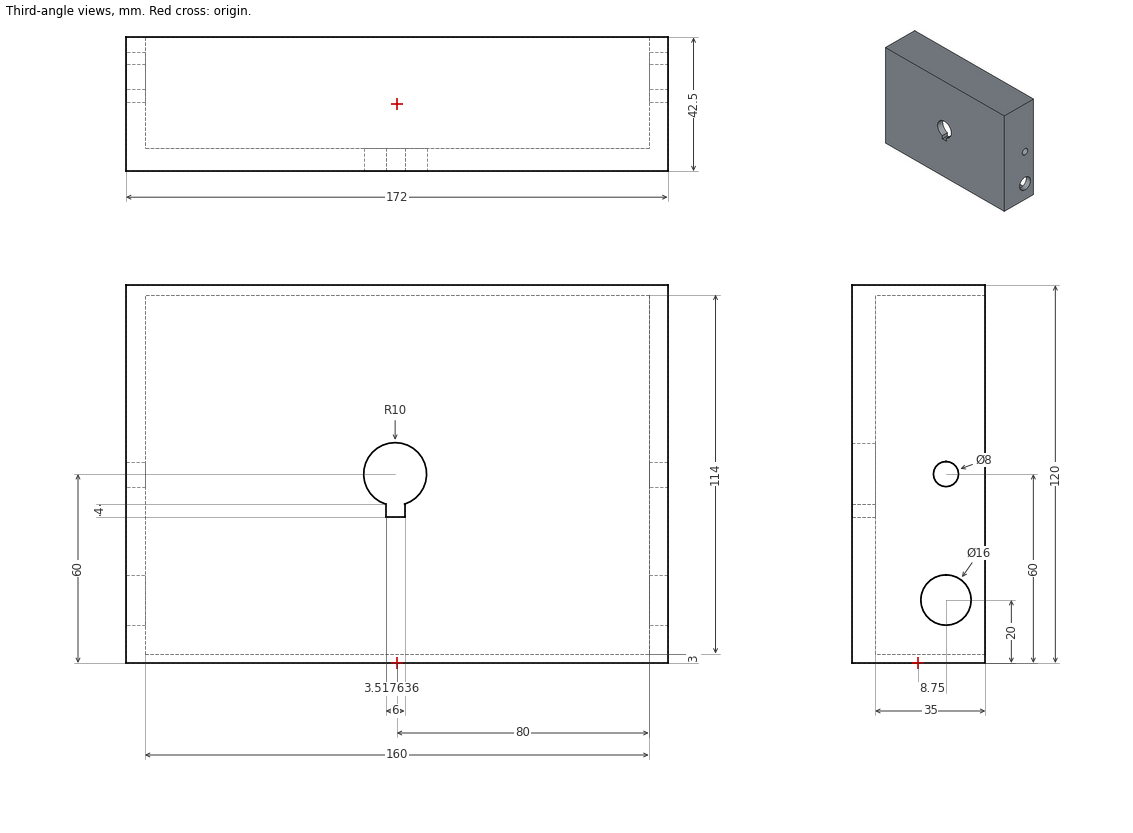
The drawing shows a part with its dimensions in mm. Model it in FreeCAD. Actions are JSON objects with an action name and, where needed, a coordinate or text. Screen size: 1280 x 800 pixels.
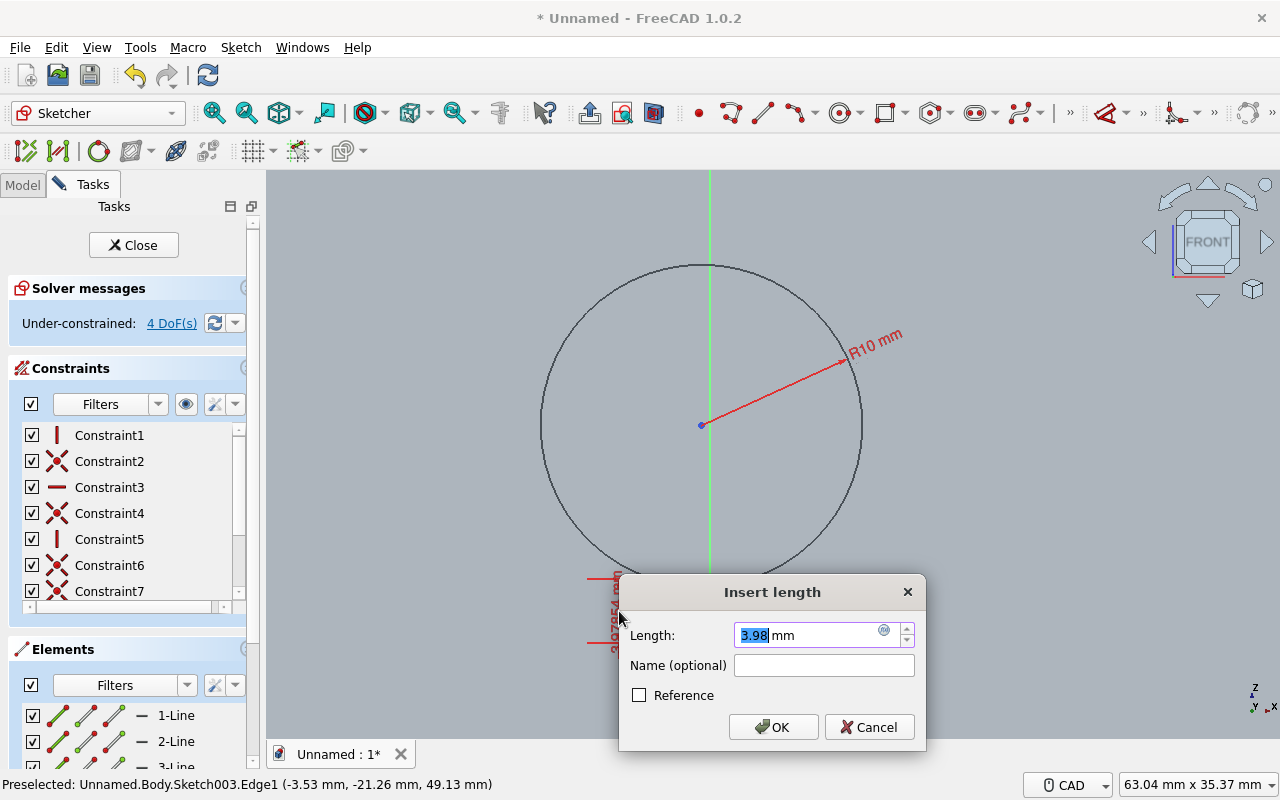
{"action": "type", "text": "4"}
{"action": "key", "text": "Return"}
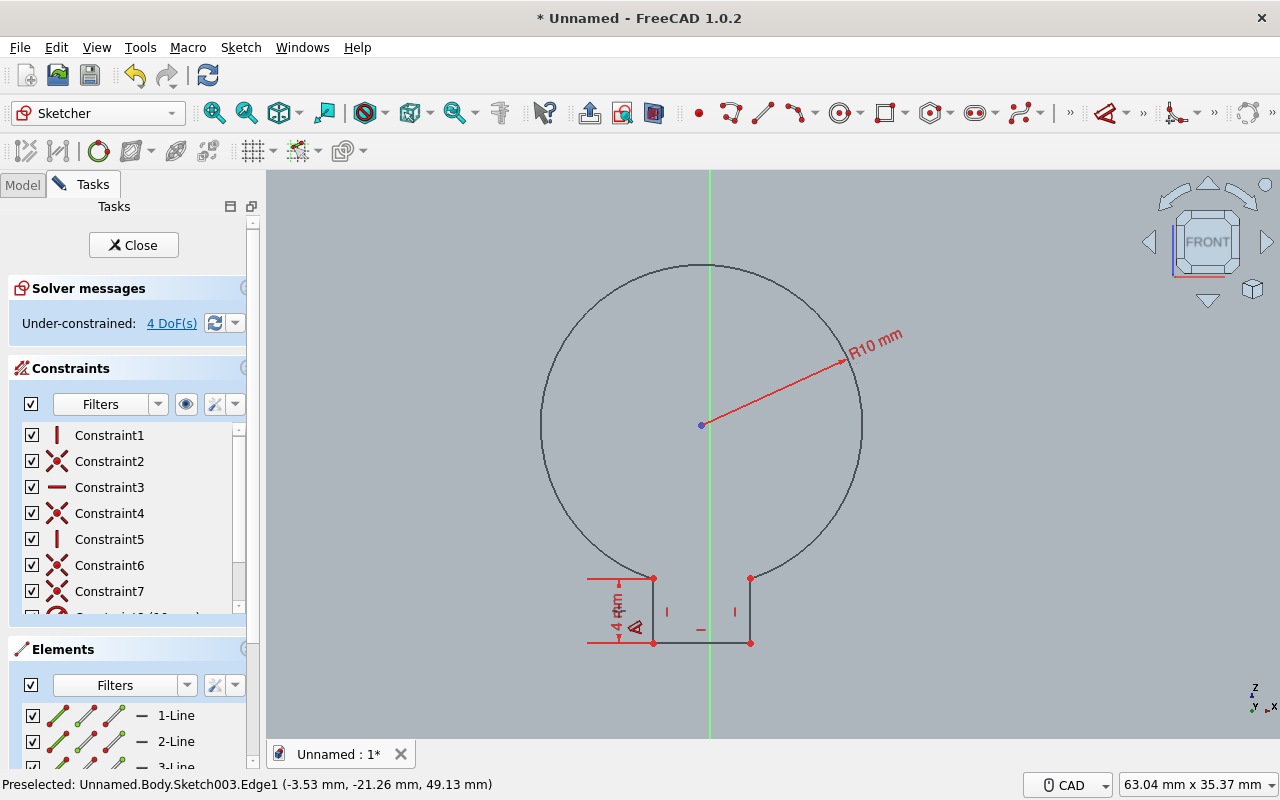
{"action": "left_click", "coordinate": [682, 643]}
{"action": "left_click", "coordinate": [679, 677]}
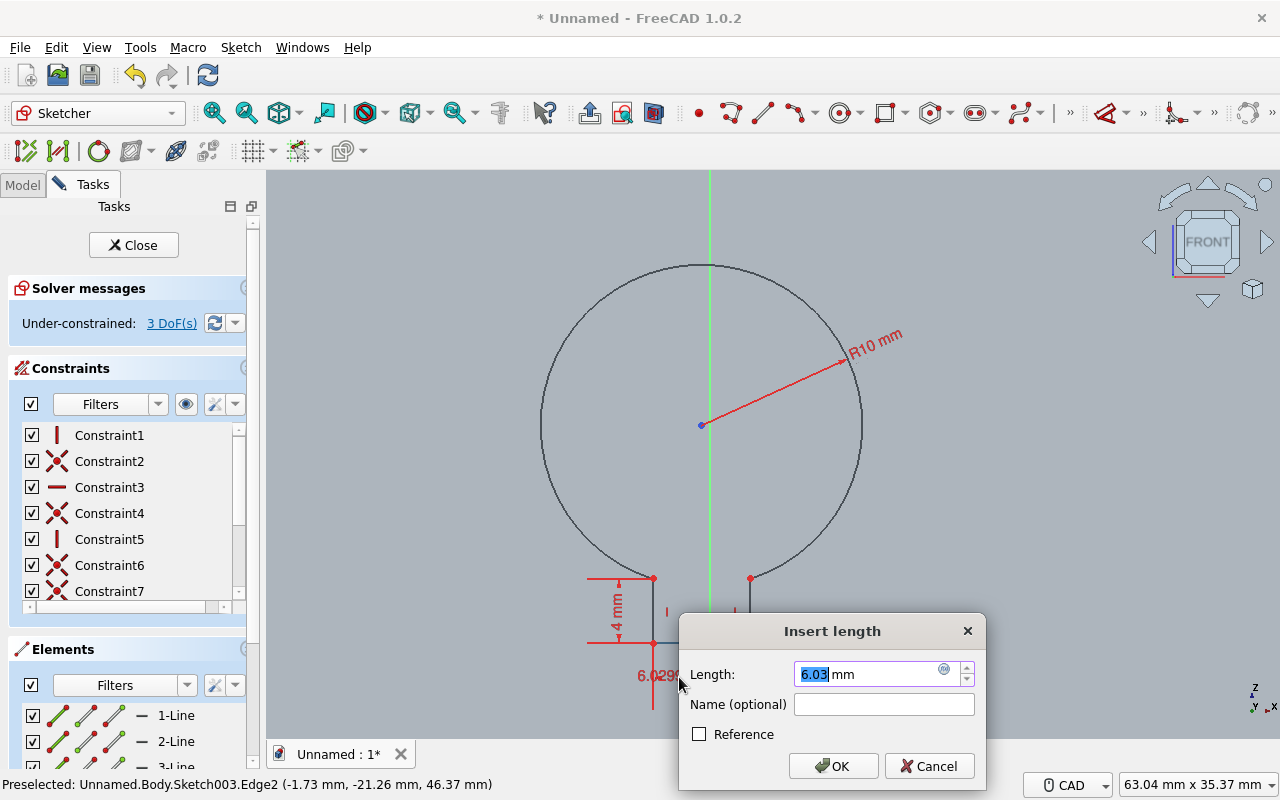
{"action": "type", "text": "6"}
{"action": "key", "text": "Return"}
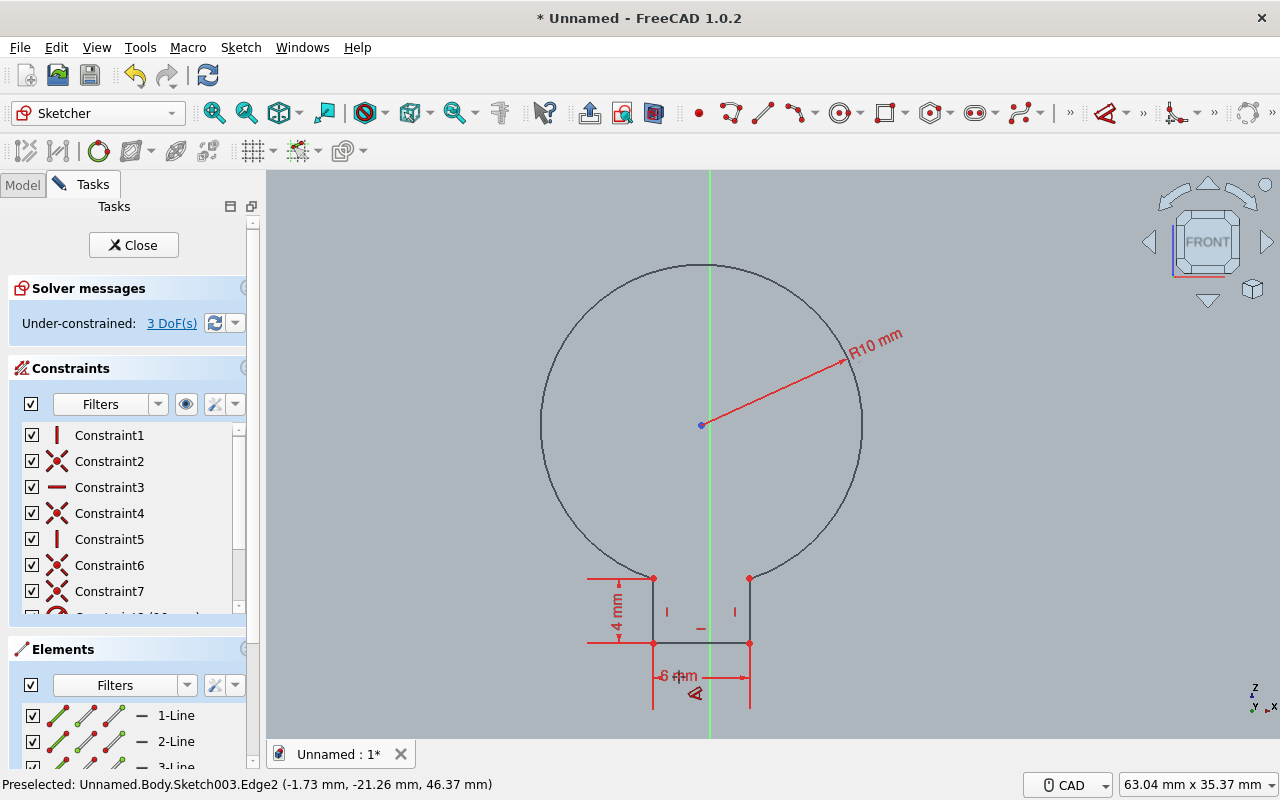
{"action": "left_click", "coordinate": [750, 624]}
{"action": "left_click", "coordinate": [784, 611]}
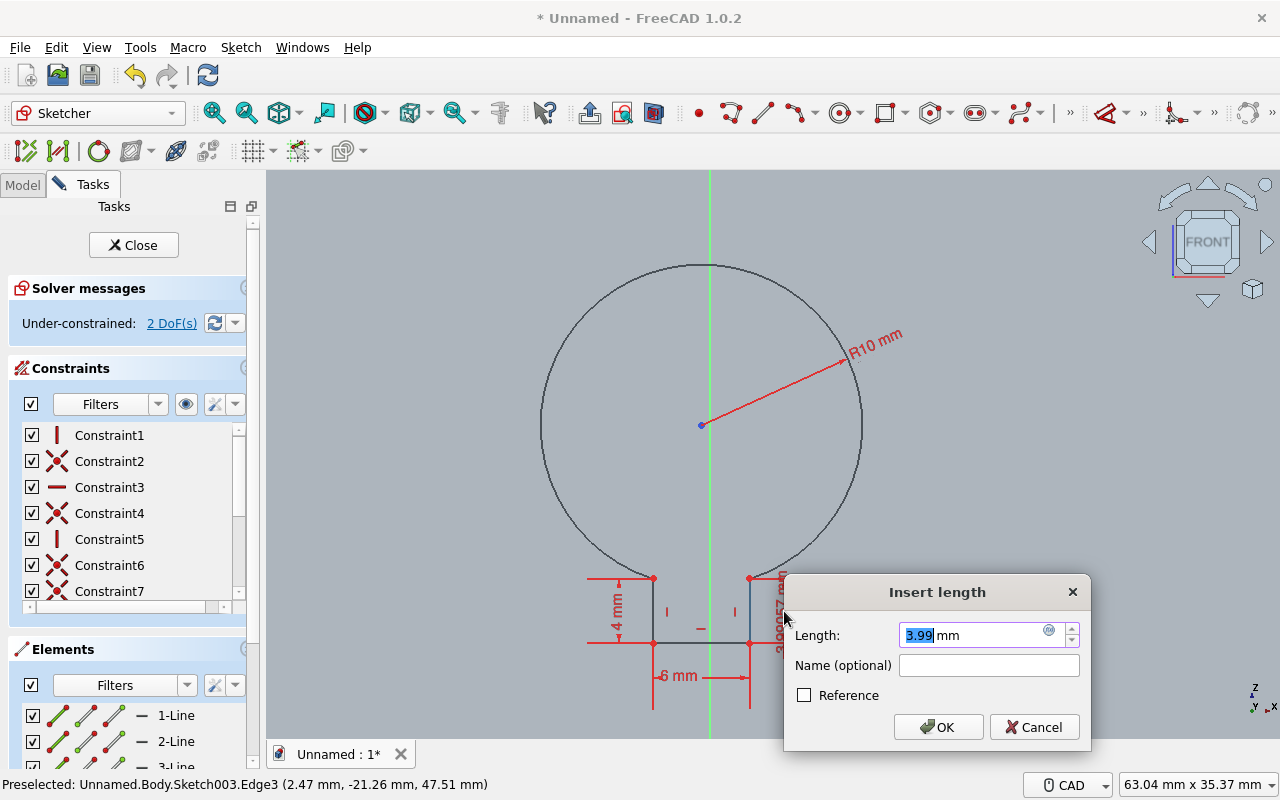
{"action": "type", "text": "4"}
{"action": "key", "text": "Return"}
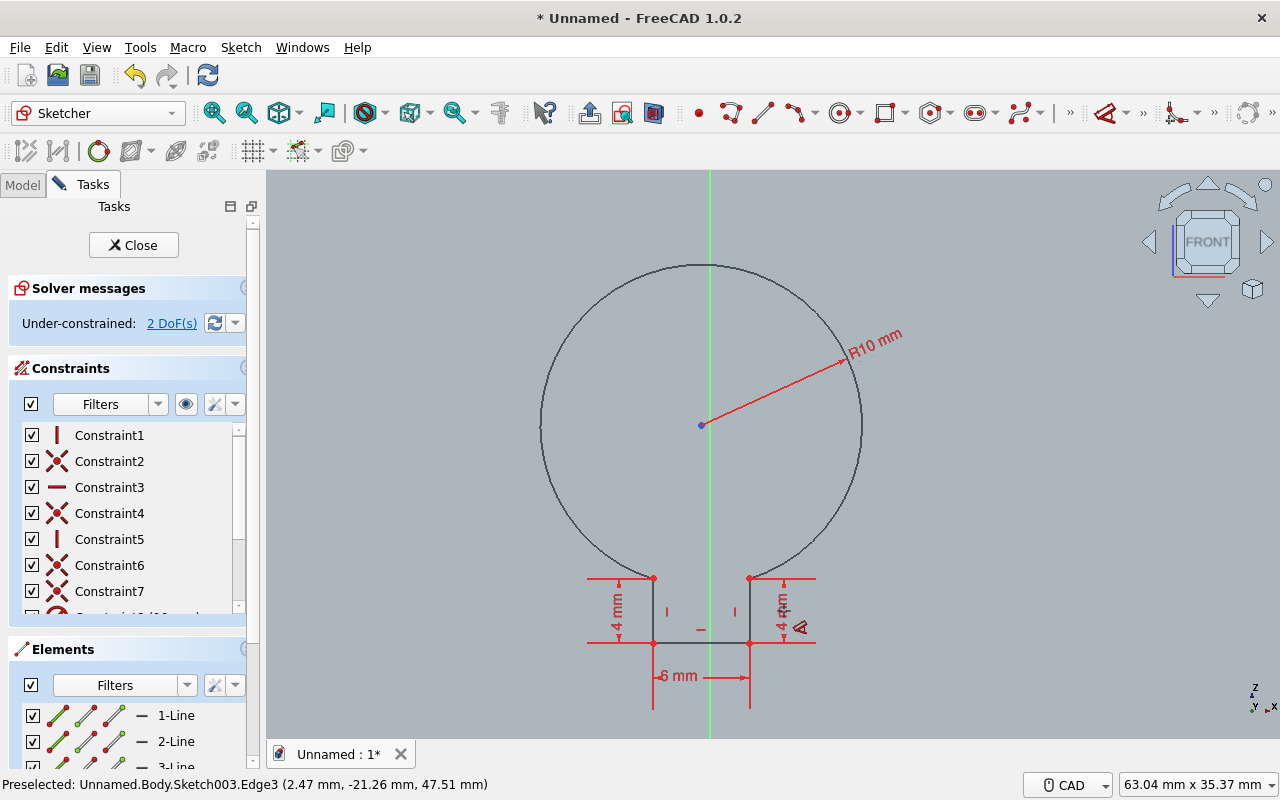
{"action": "left_click", "coordinate": [701, 425]}
{"action": "left_click", "coordinate": [744, 503]}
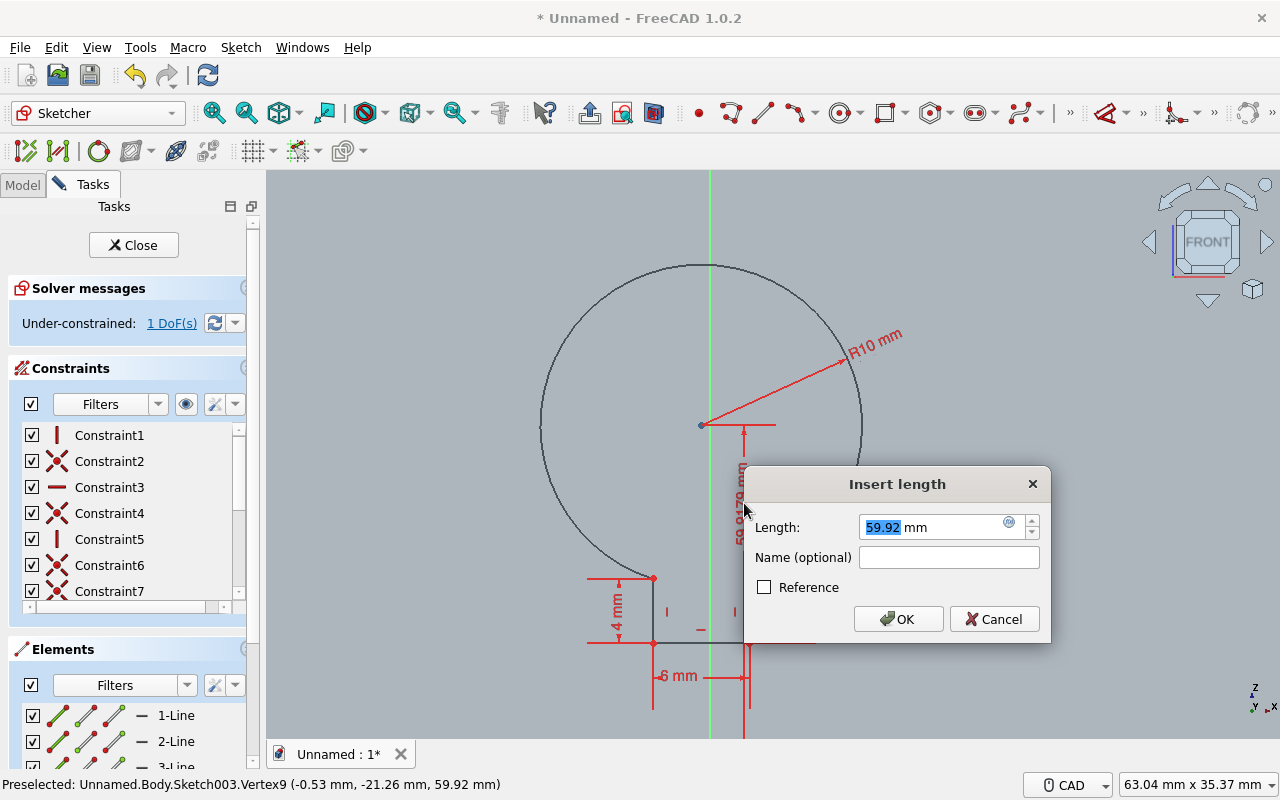
{"action": "type", "text": "60"}
{"action": "key", "text": "Return"}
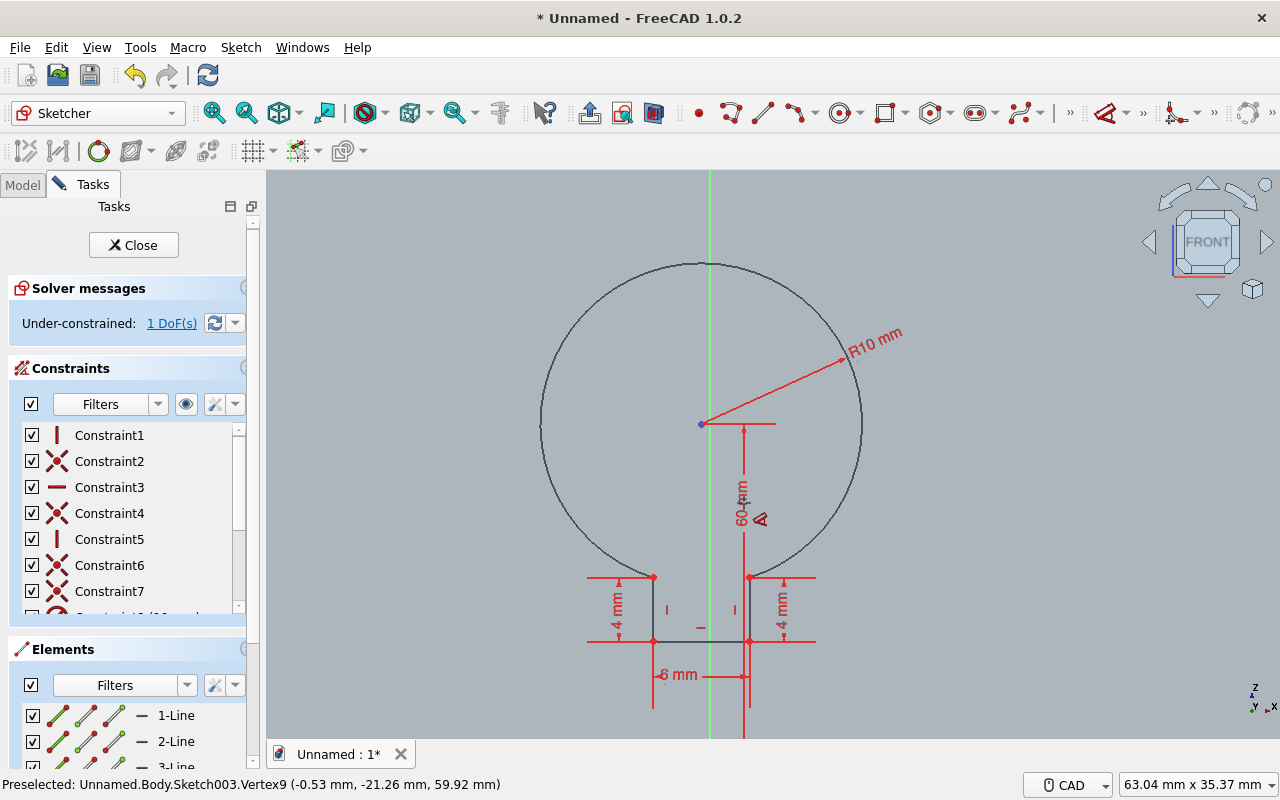
{"action": "left_click", "coordinate": [653, 578]}
{"action": "left_click", "coordinate": [681, 544]}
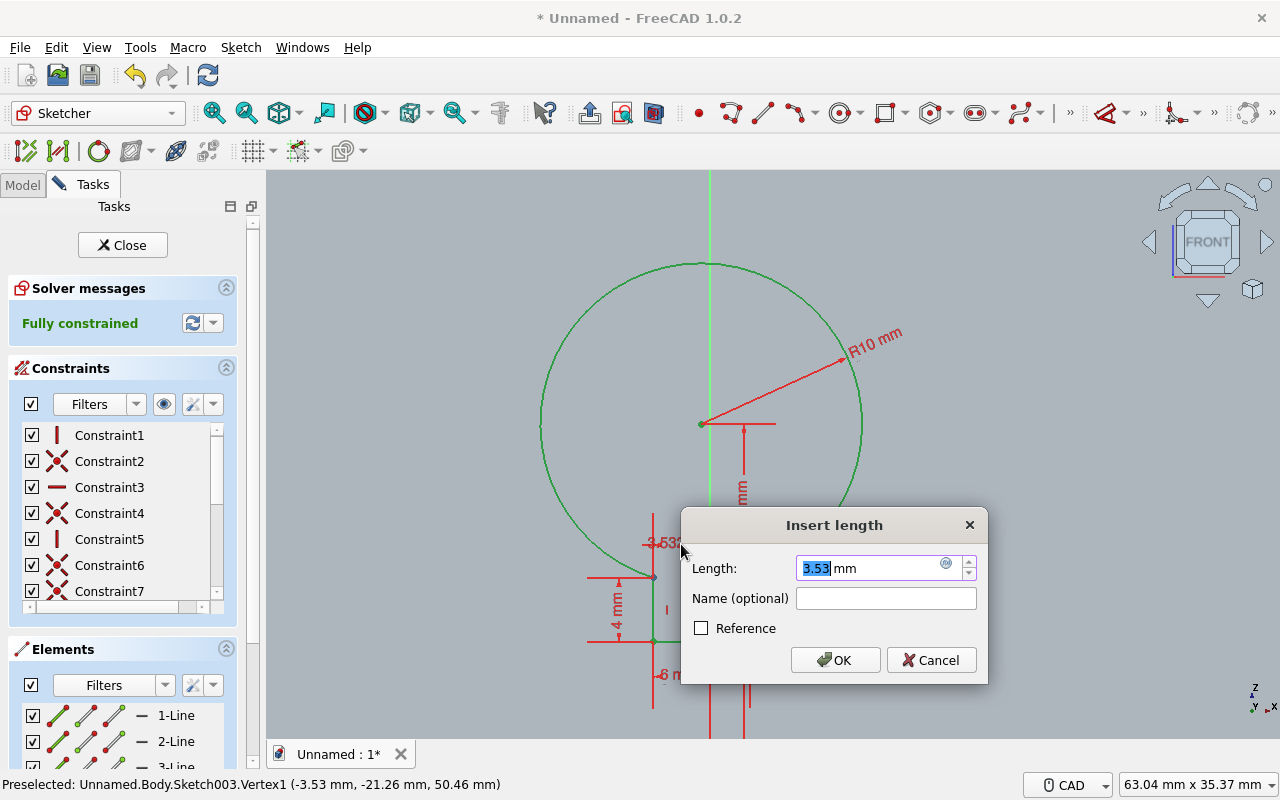
{"action": "type", "text": "3.517636"}
{"action": "key", "text": "Return"}
{"action": "key", "text": "Escape"}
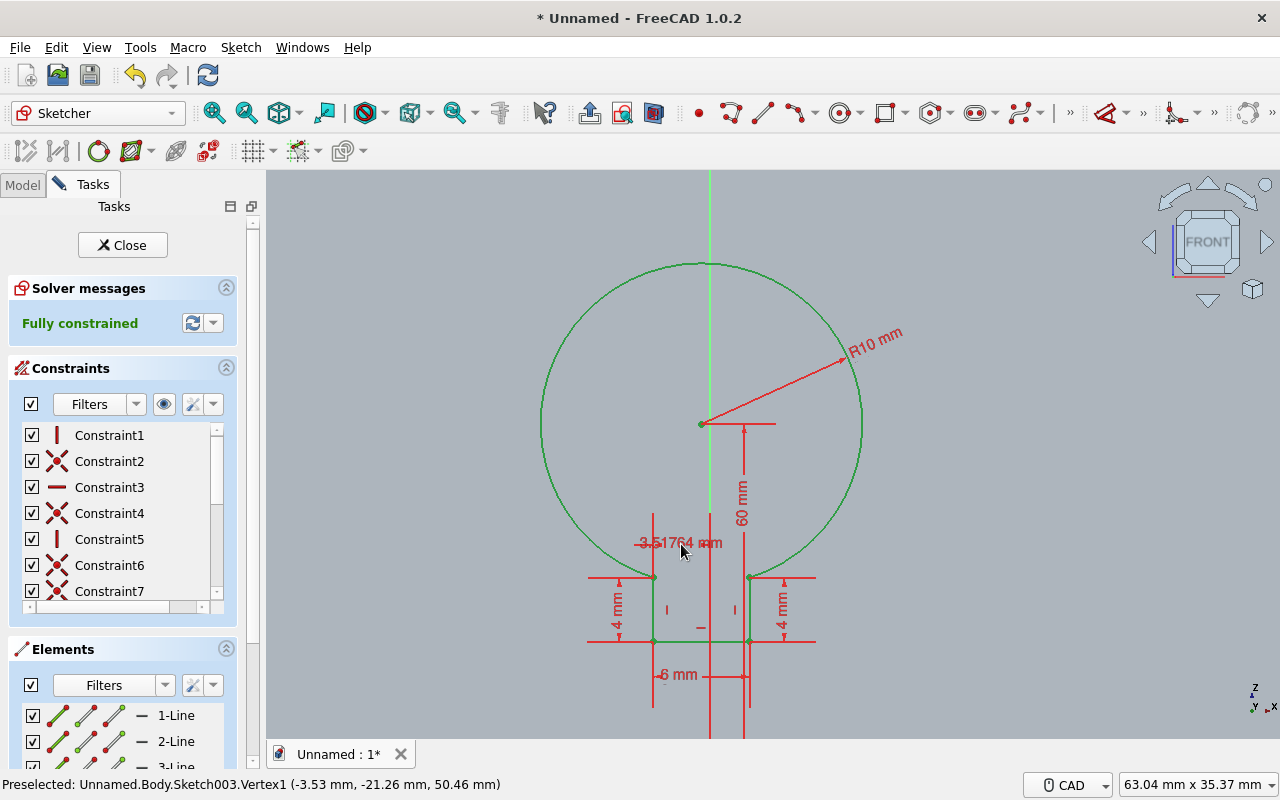
{"action": "left_click", "coordinate": [123, 245]}